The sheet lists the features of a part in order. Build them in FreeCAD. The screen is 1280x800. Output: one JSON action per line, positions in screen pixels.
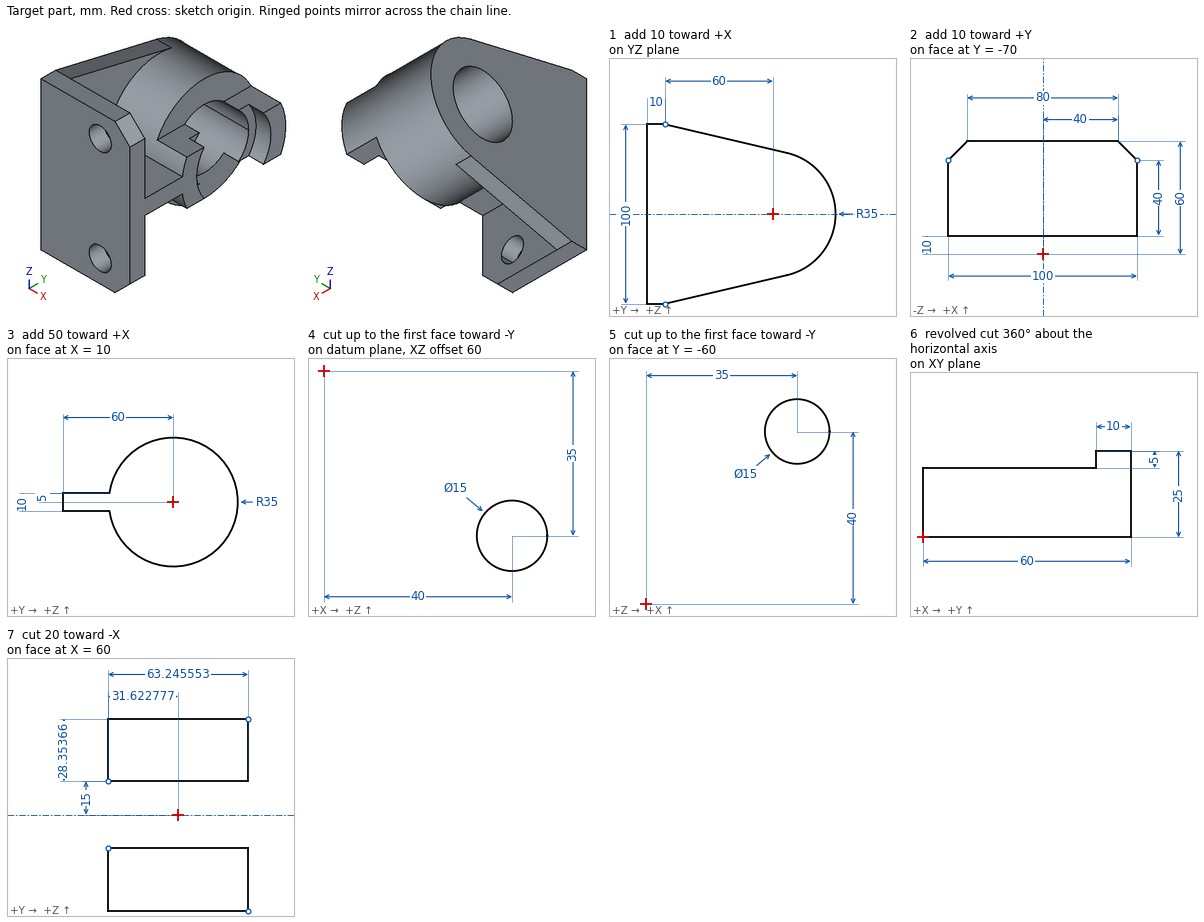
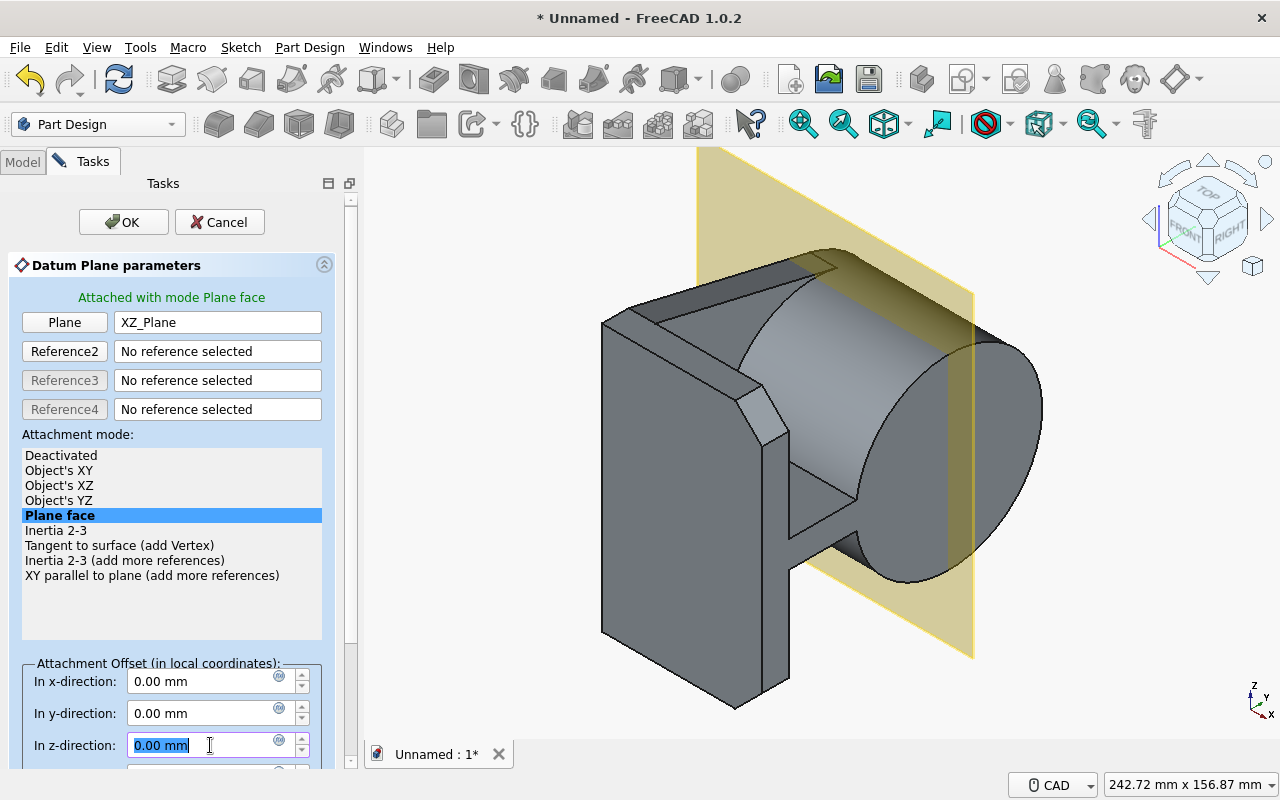
{"action": "type", "text": "60"}
{"action": "key", "text": "Tab"}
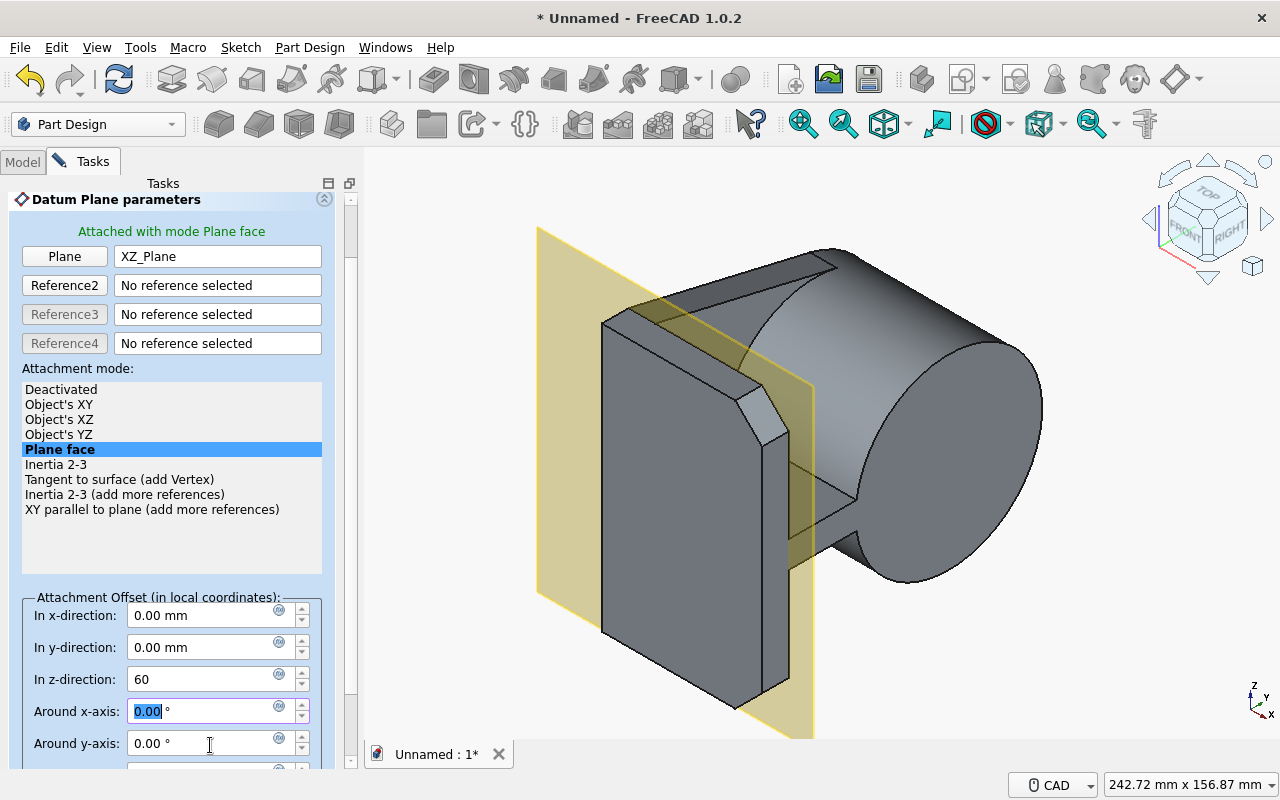
{"action": "scroll", "coordinate": [351, 480], "scroll_direction": "up", "scroll_amount": 2}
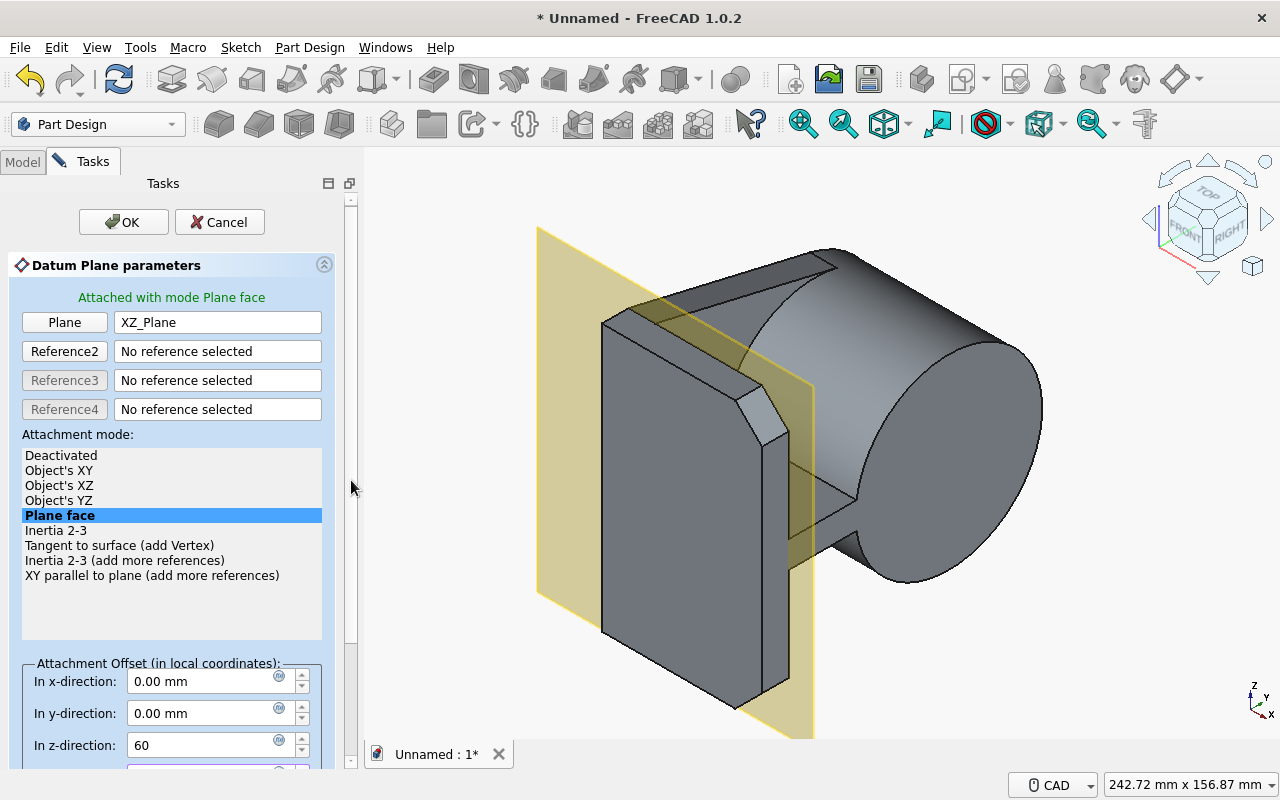
{"action": "left_click", "coordinate": [124, 222]}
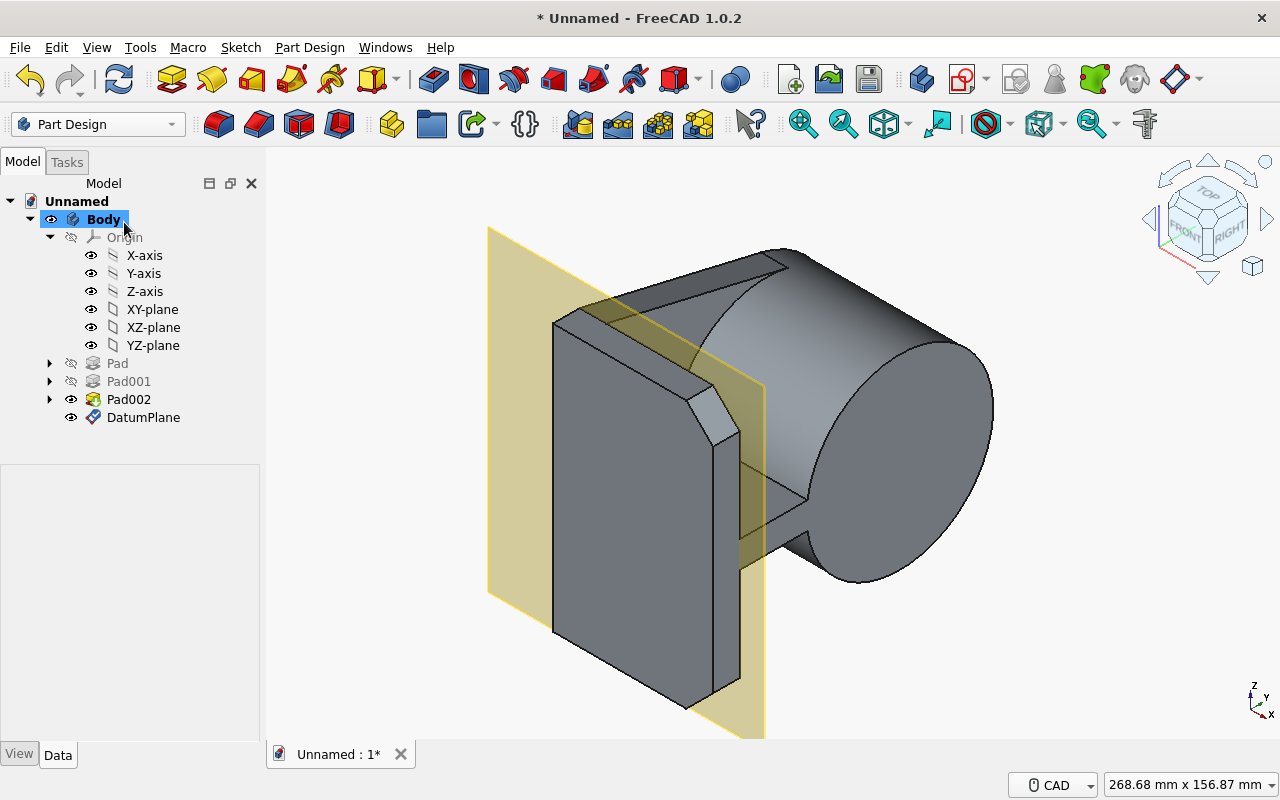
{"action": "left_click", "coordinate": [116, 417]}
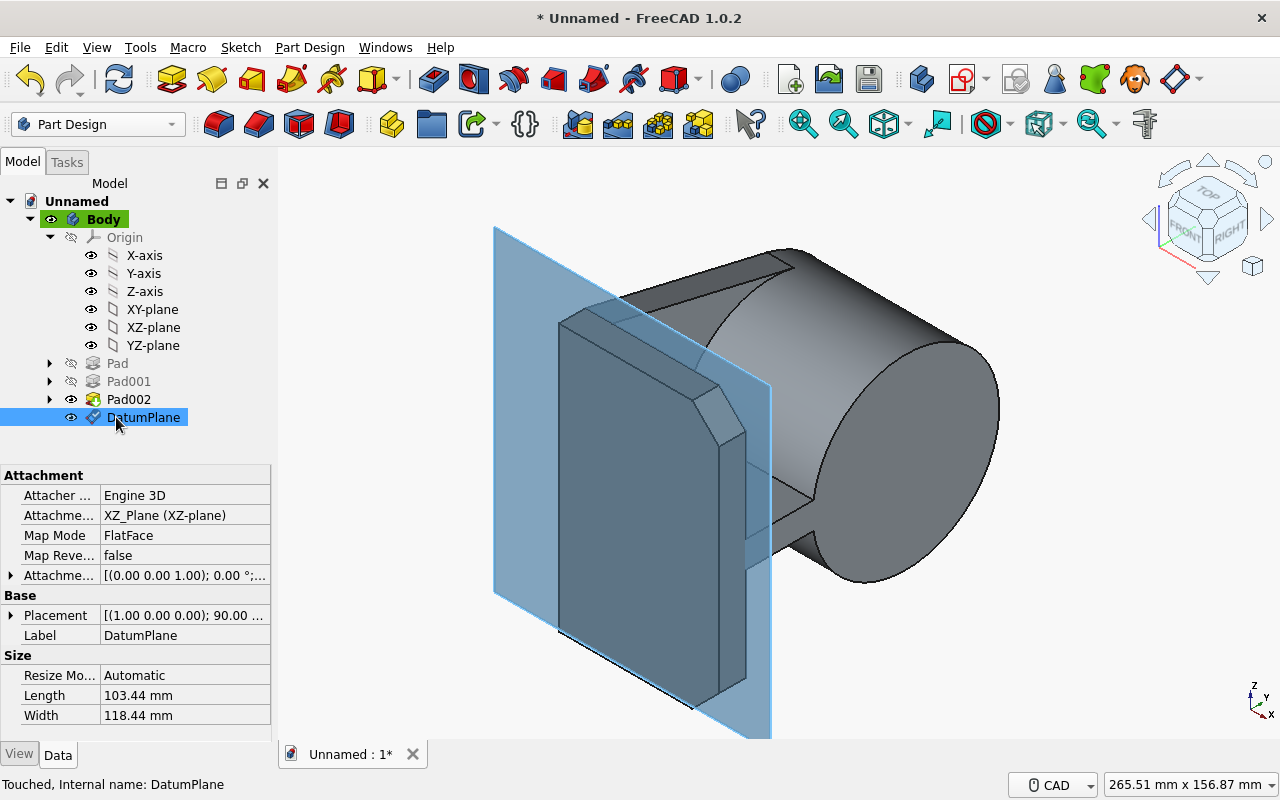
{"action": "left_click", "coordinate": [962, 80]}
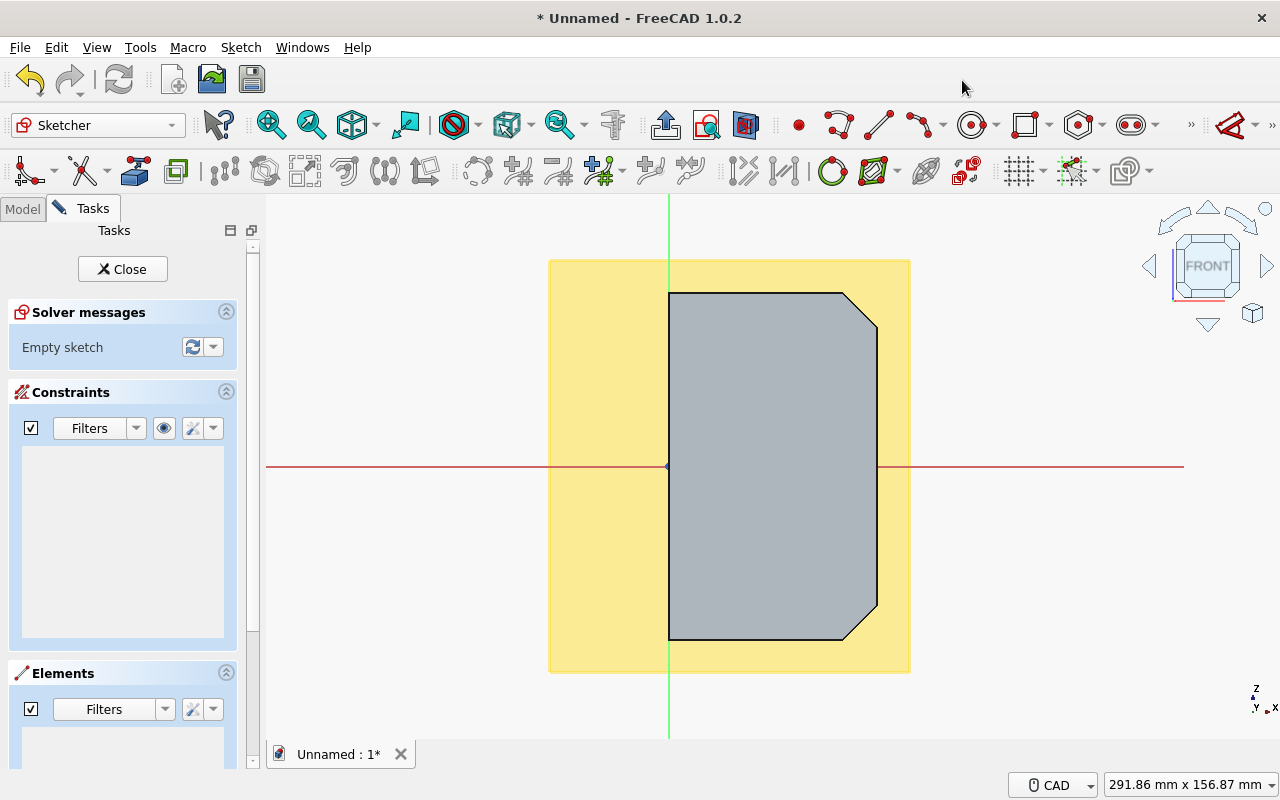
{"action": "left_click", "coordinate": [746, 126]}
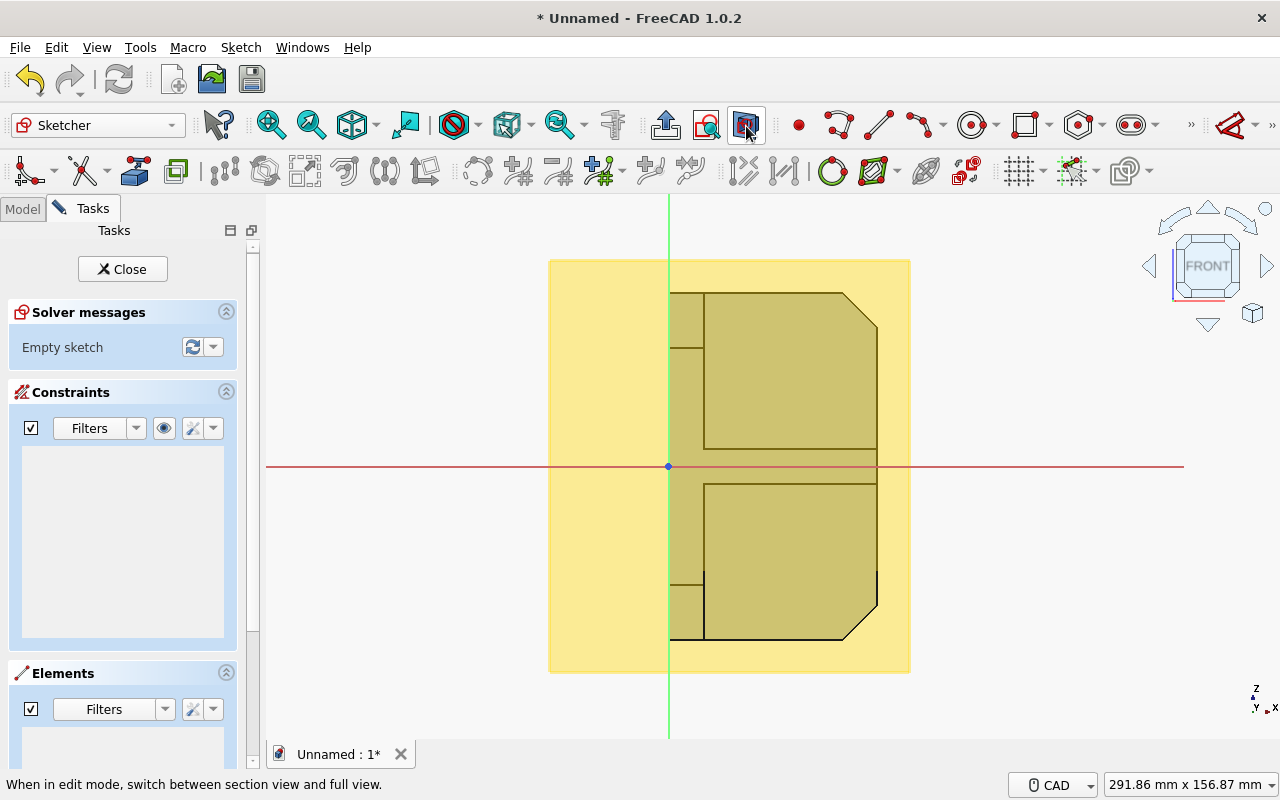
{"action": "scroll", "coordinate": [828, 612], "scroll_direction": "up", "scroll_amount": 9}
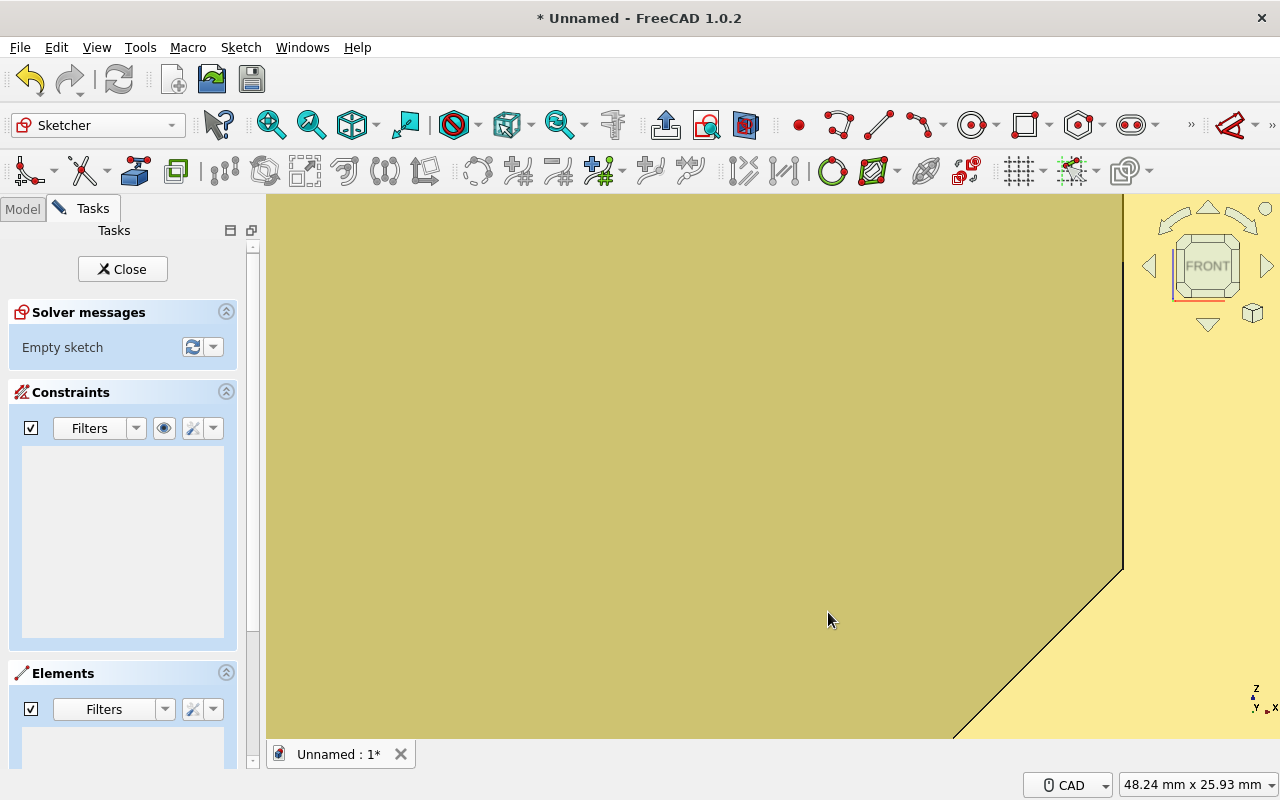
{"action": "key", "text": "g c"}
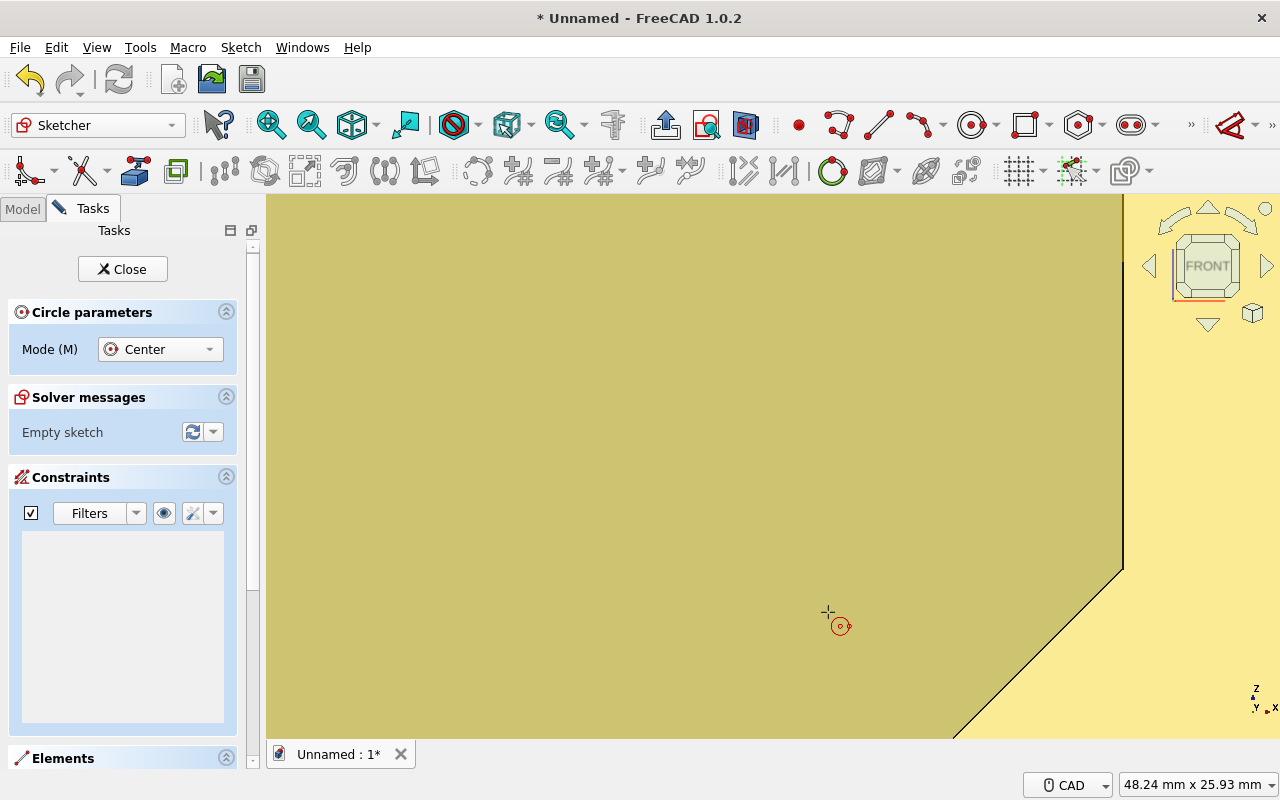
{"action": "left_click", "coordinate": [703, 464]}
{"action": "left_click", "coordinate": [814, 352]}
{"action": "key", "text": "Escape"}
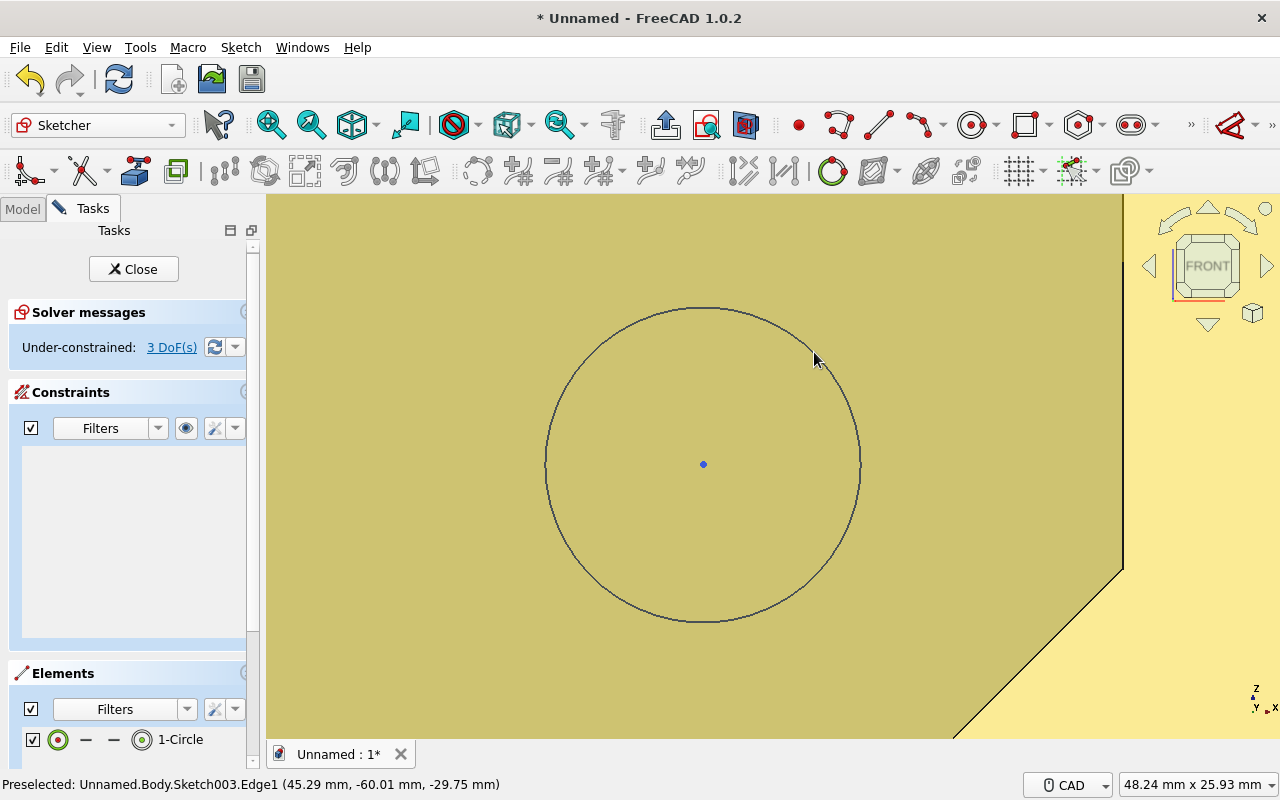
{"action": "left_click", "coordinate": [1230, 126]}